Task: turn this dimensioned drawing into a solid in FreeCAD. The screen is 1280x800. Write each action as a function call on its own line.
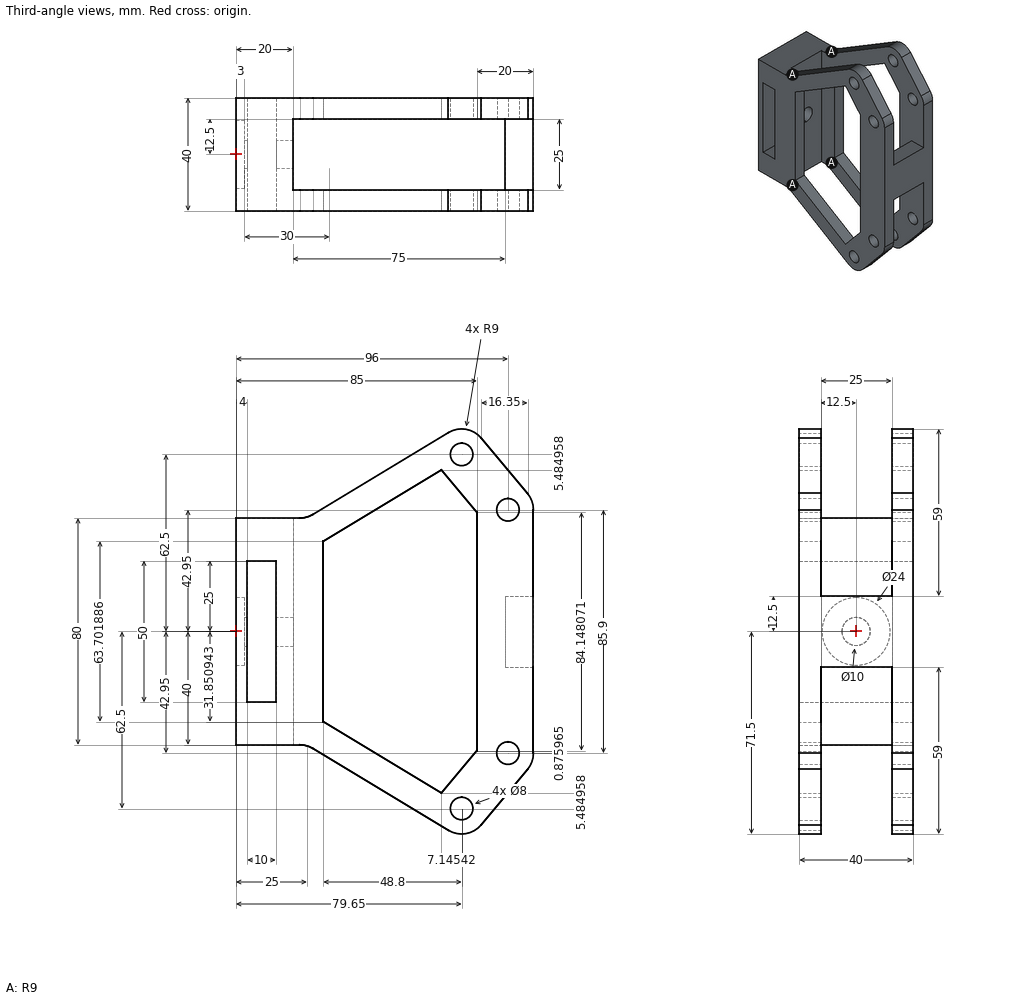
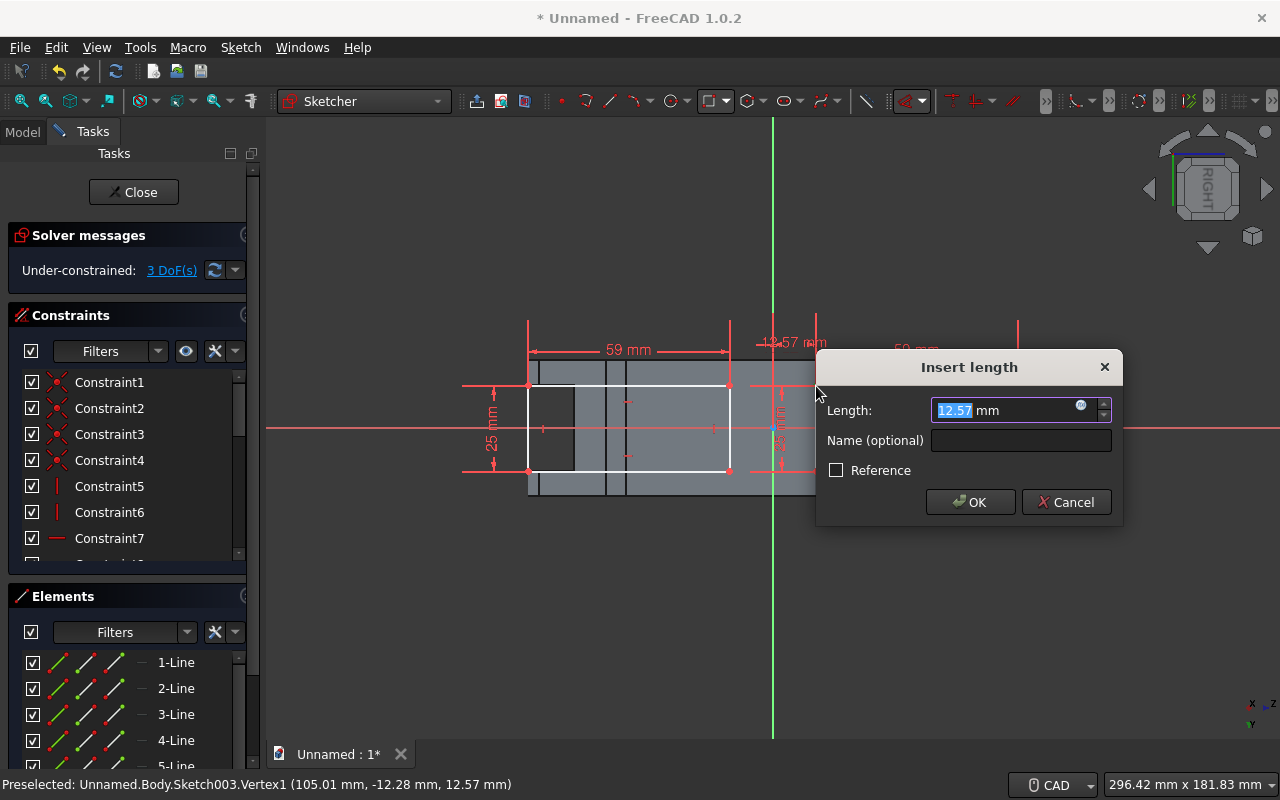
text(12.5)
key(Return)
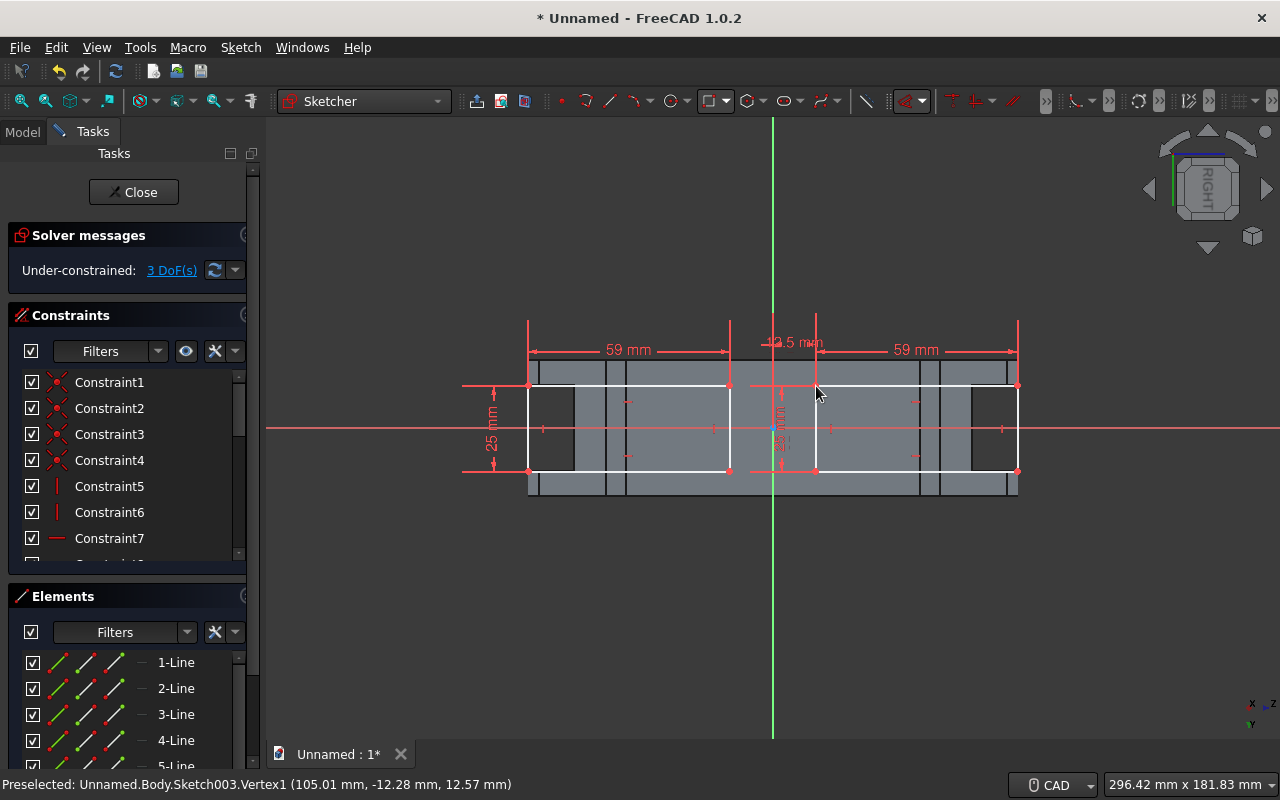
click(816, 386)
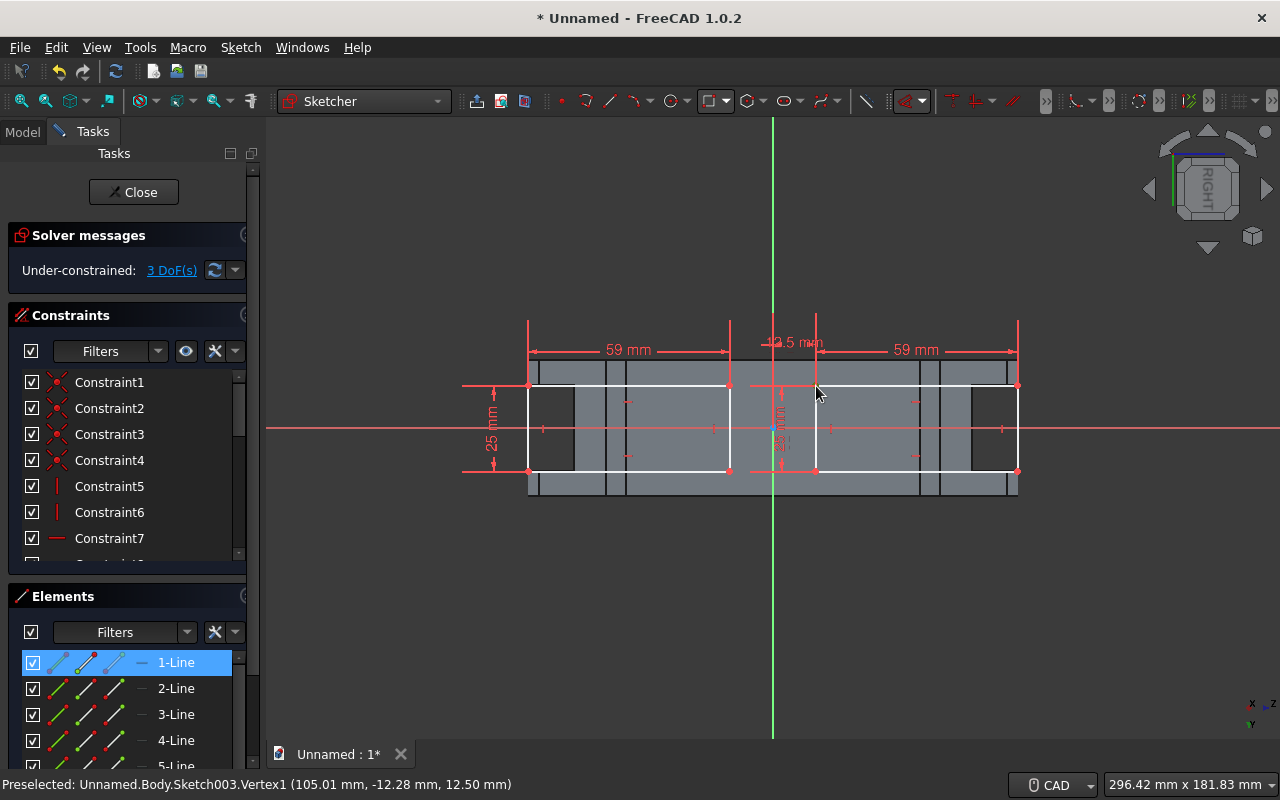
key(i)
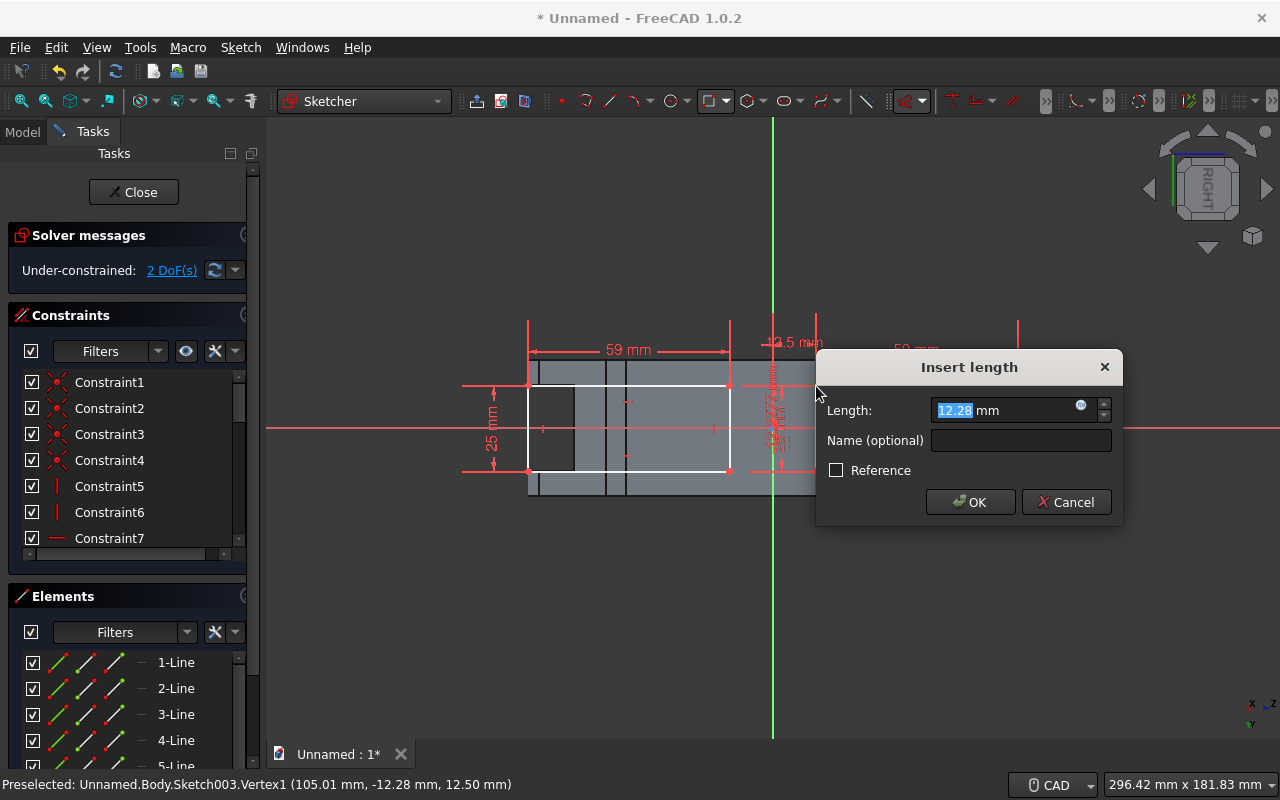
text(12.5)
key(Return)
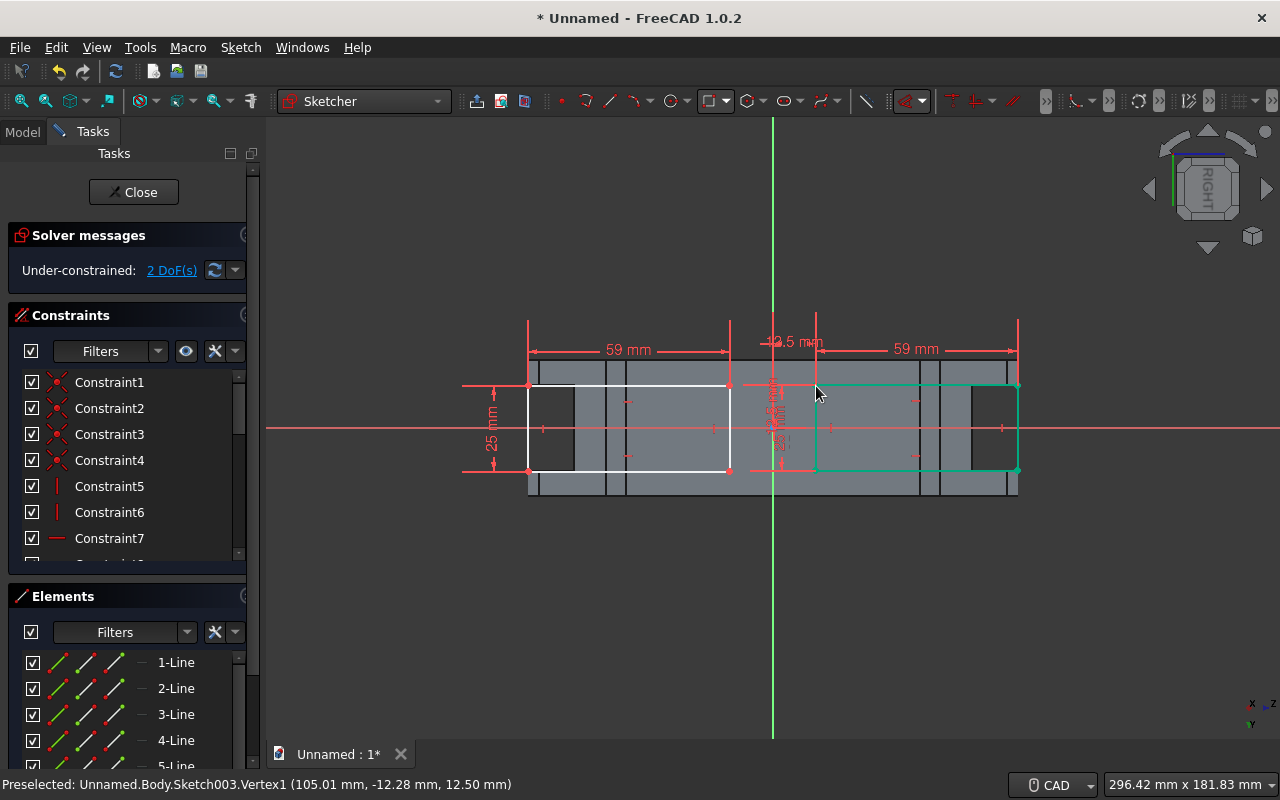
click(528, 386)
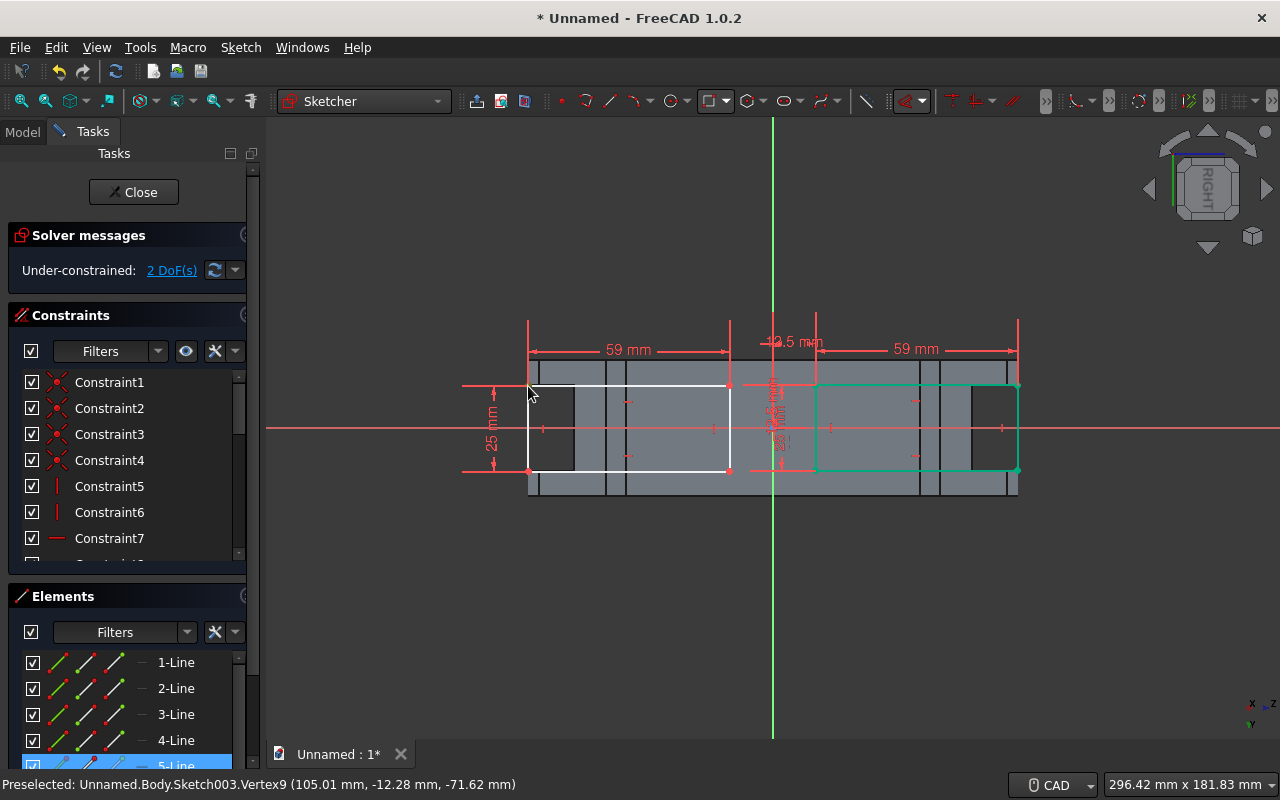
key(l)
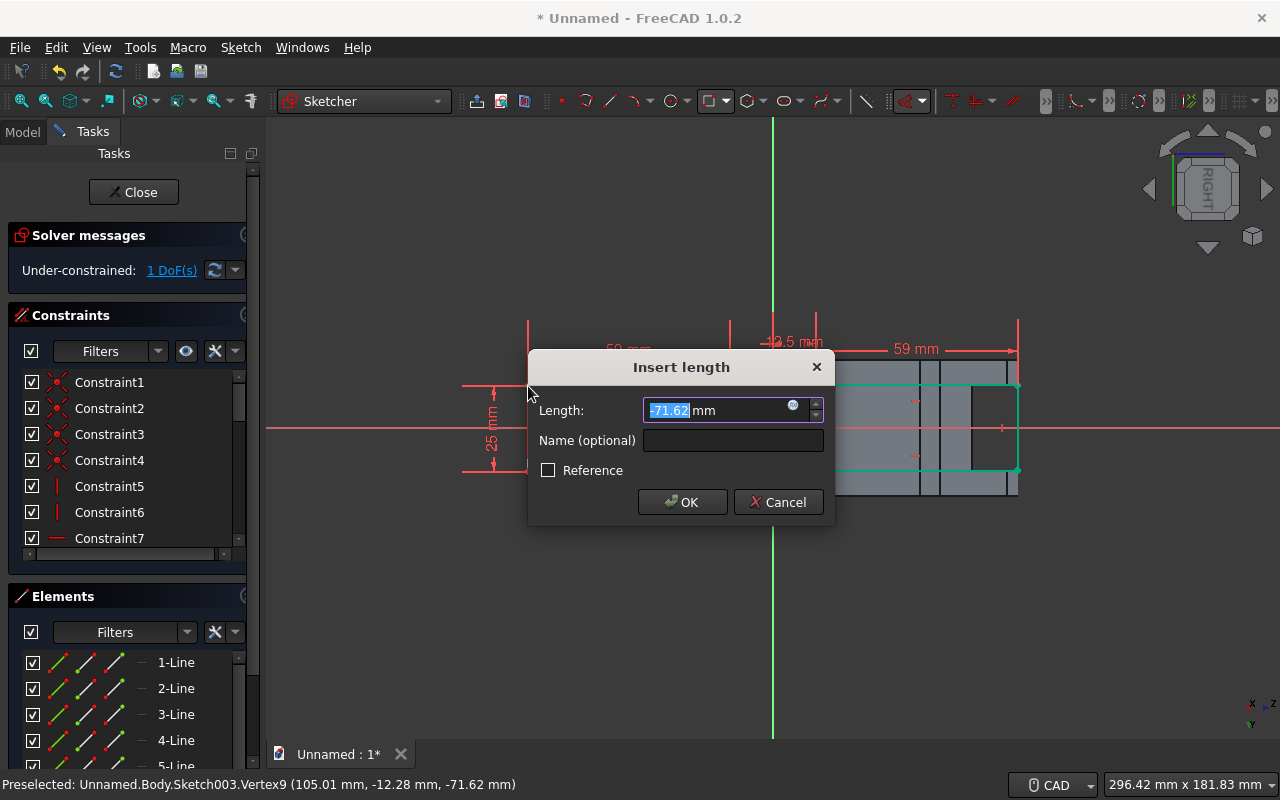
text(-71.5)
key(Return)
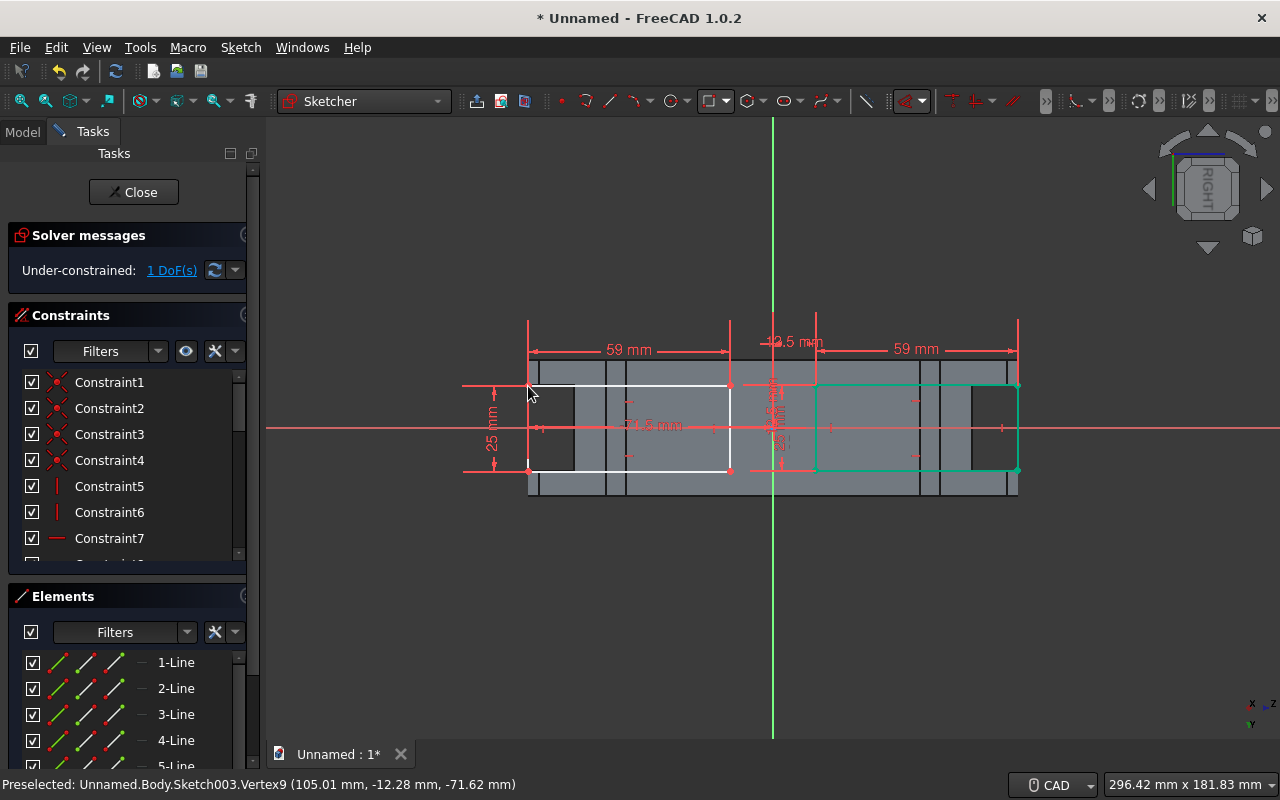
click(528, 386)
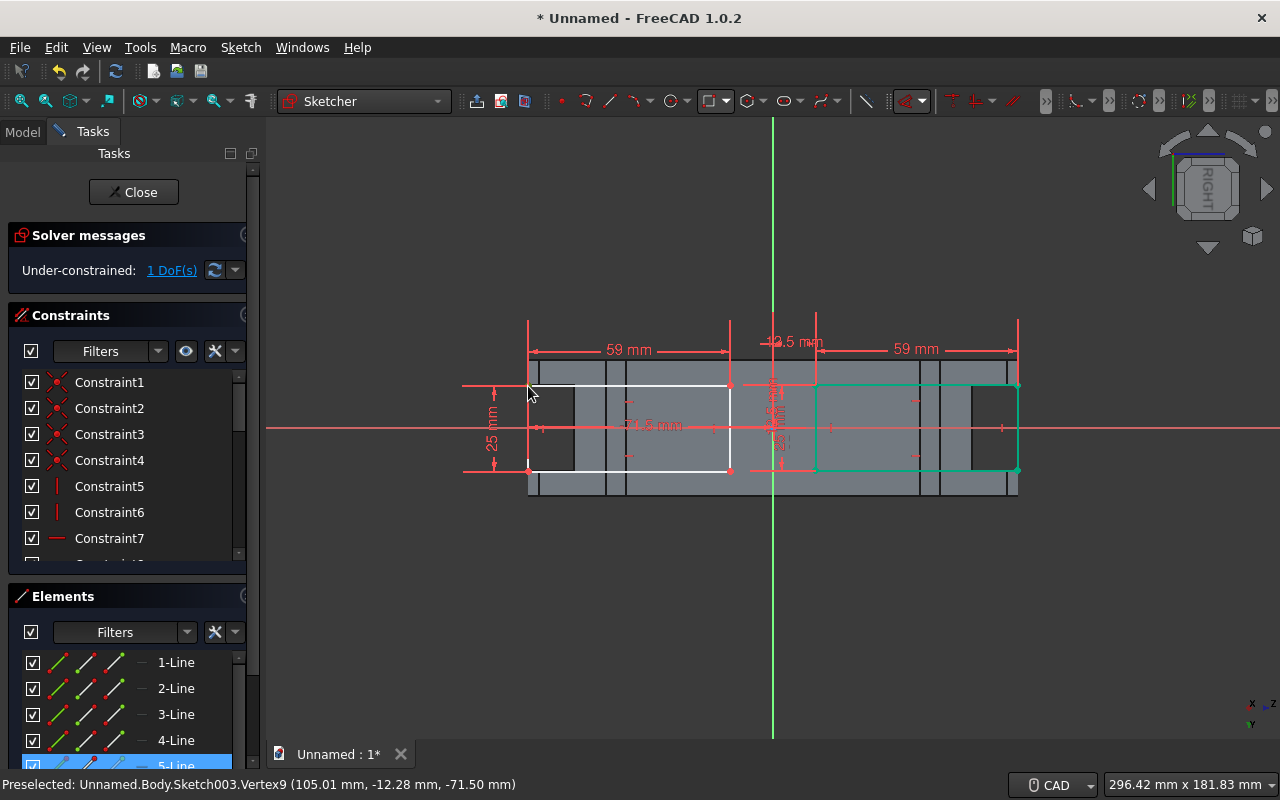
key(i)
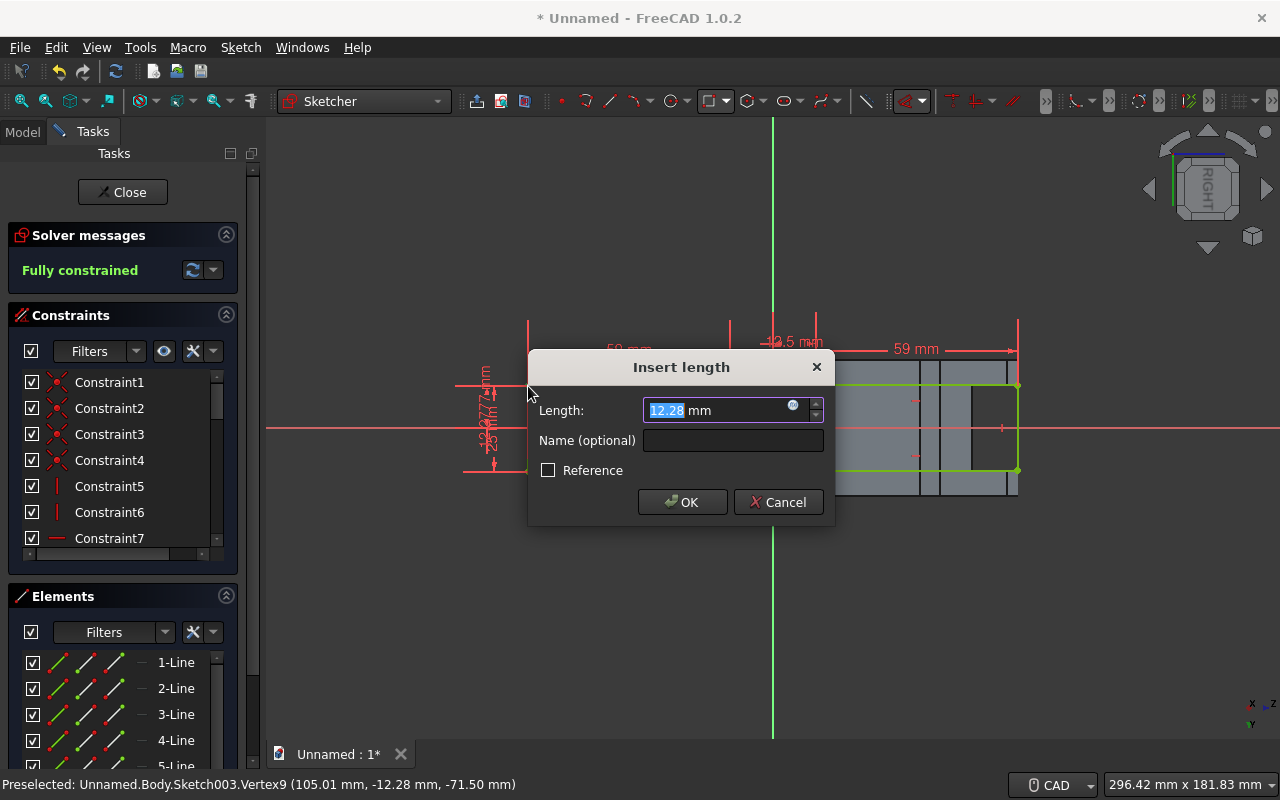
text(12.5)
key(Return)